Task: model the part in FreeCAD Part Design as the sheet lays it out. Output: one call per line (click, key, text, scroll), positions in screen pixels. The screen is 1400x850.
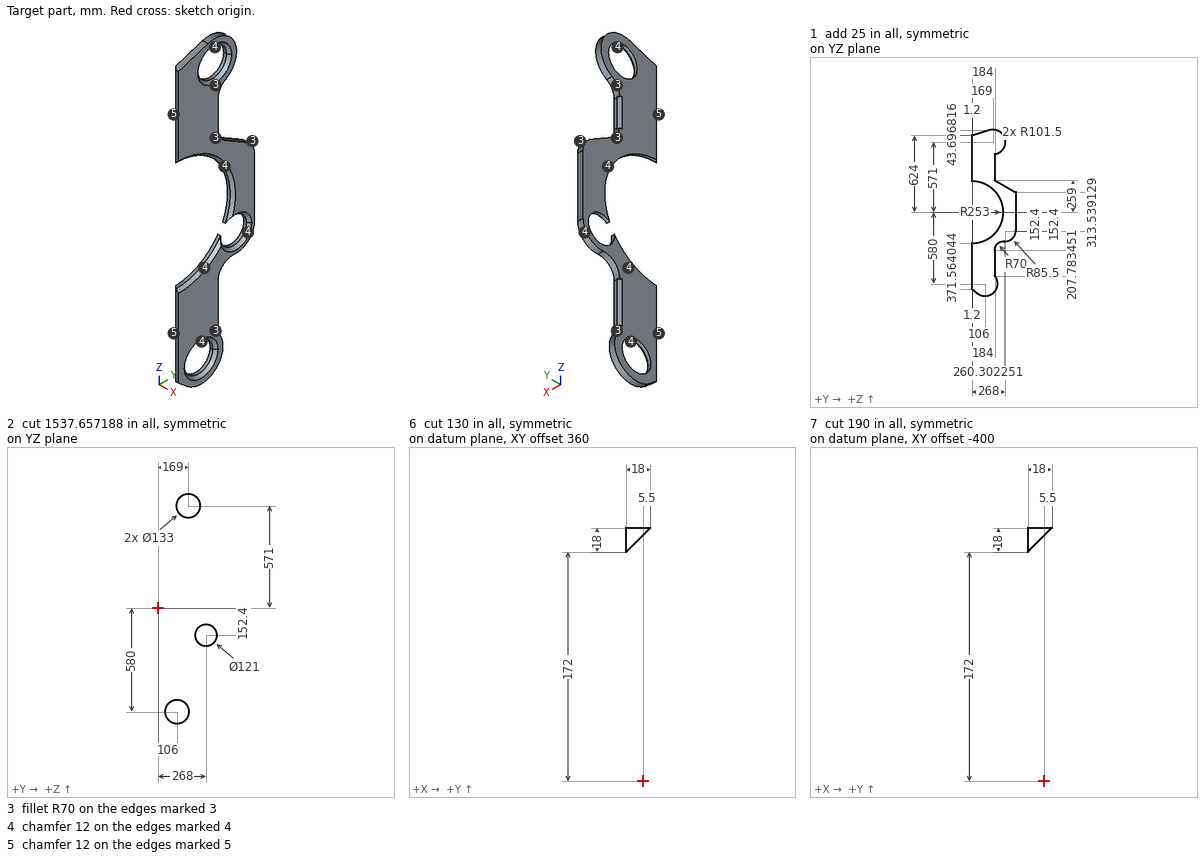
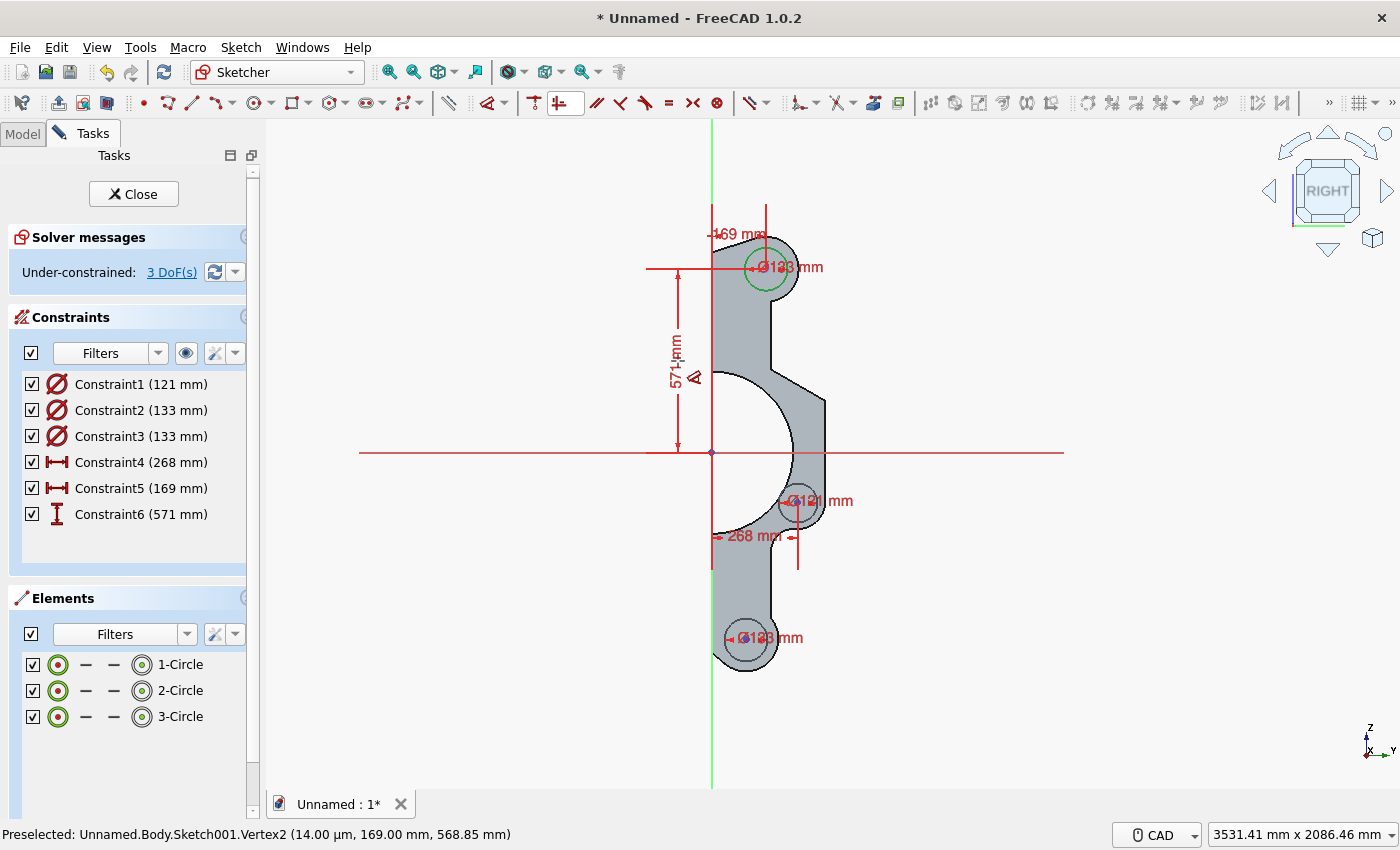
click(746, 640)
click(729, 674)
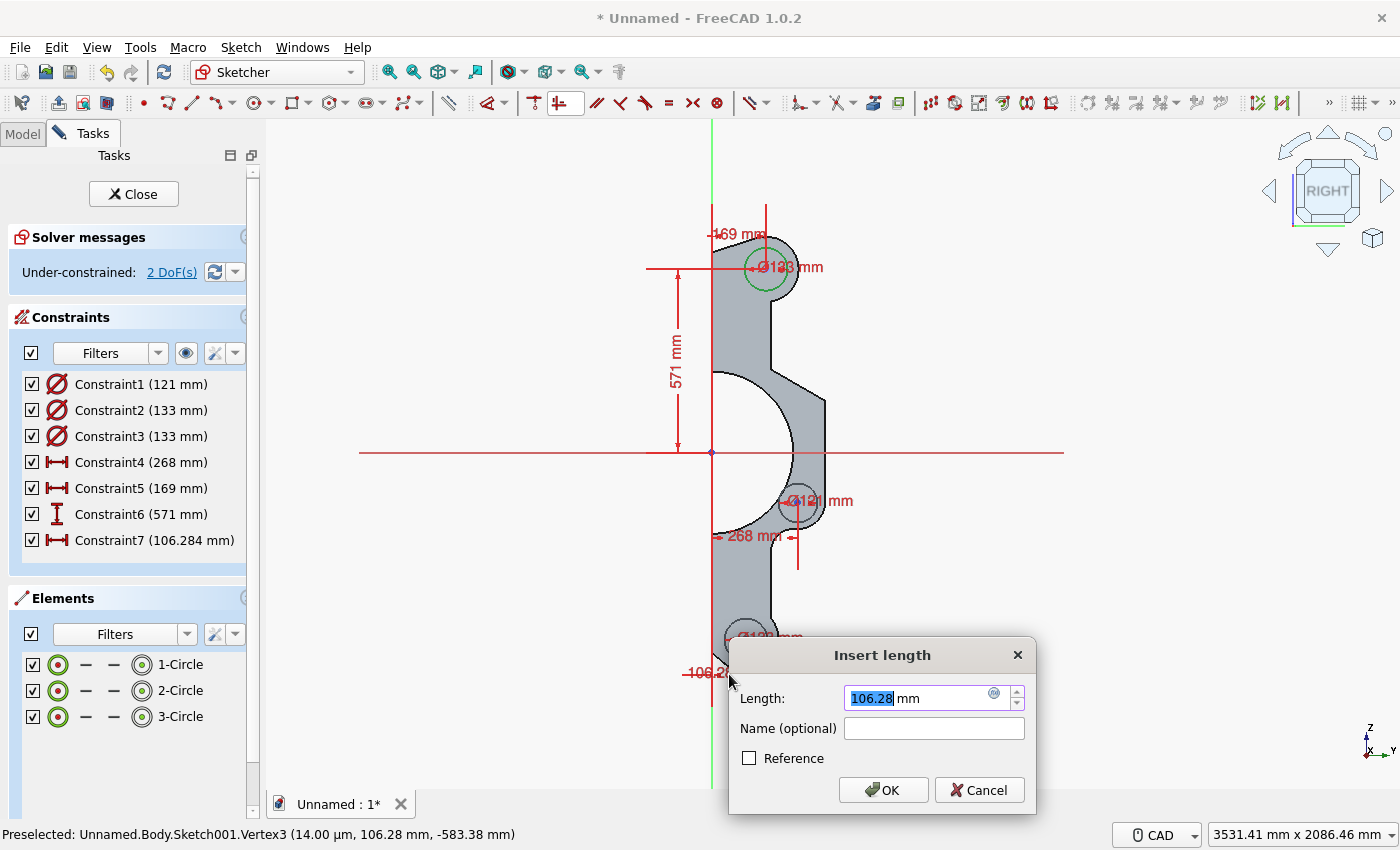
text(106)
key(Return)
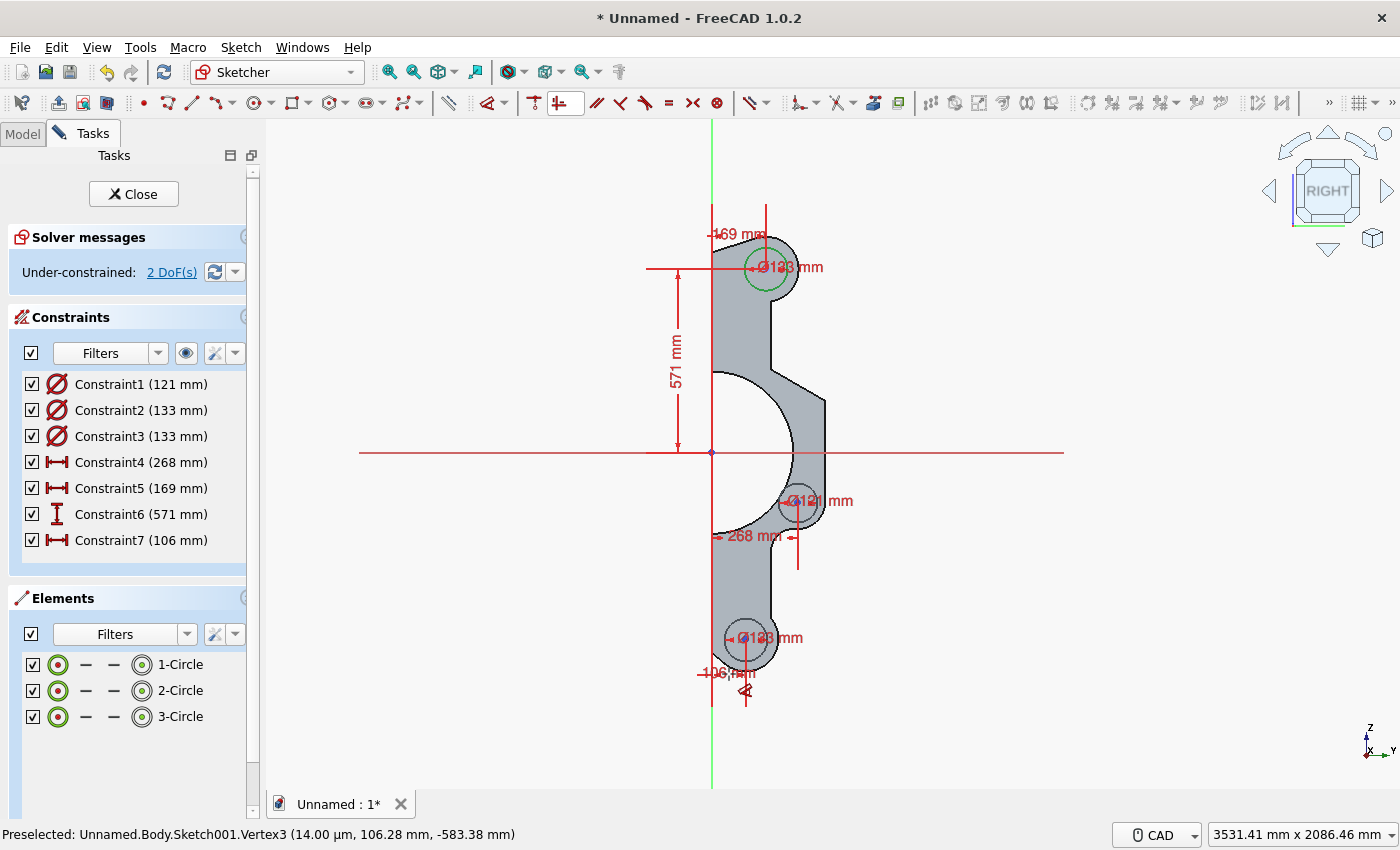
click(746, 640)
click(678, 546)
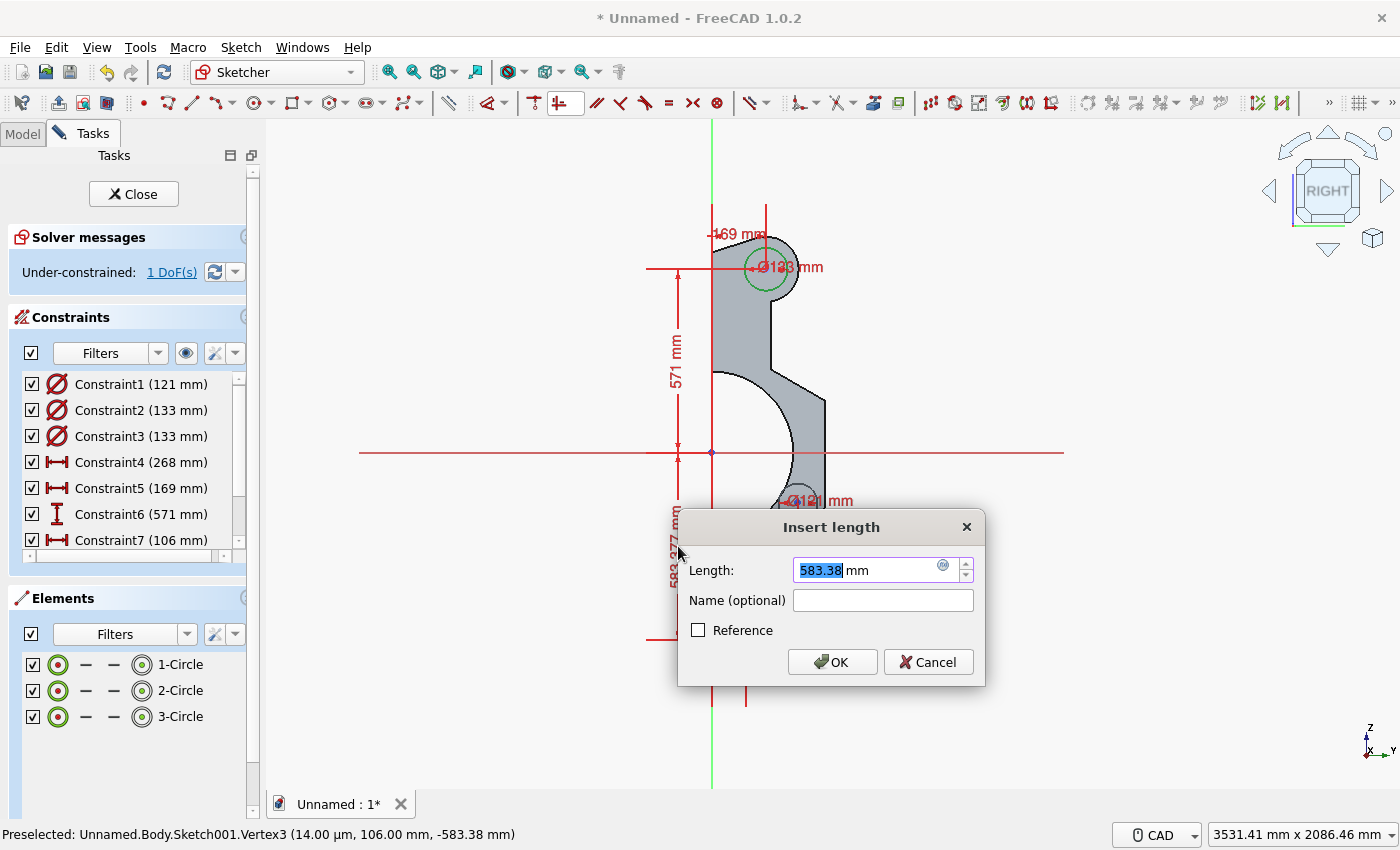
text(580)
key(Return)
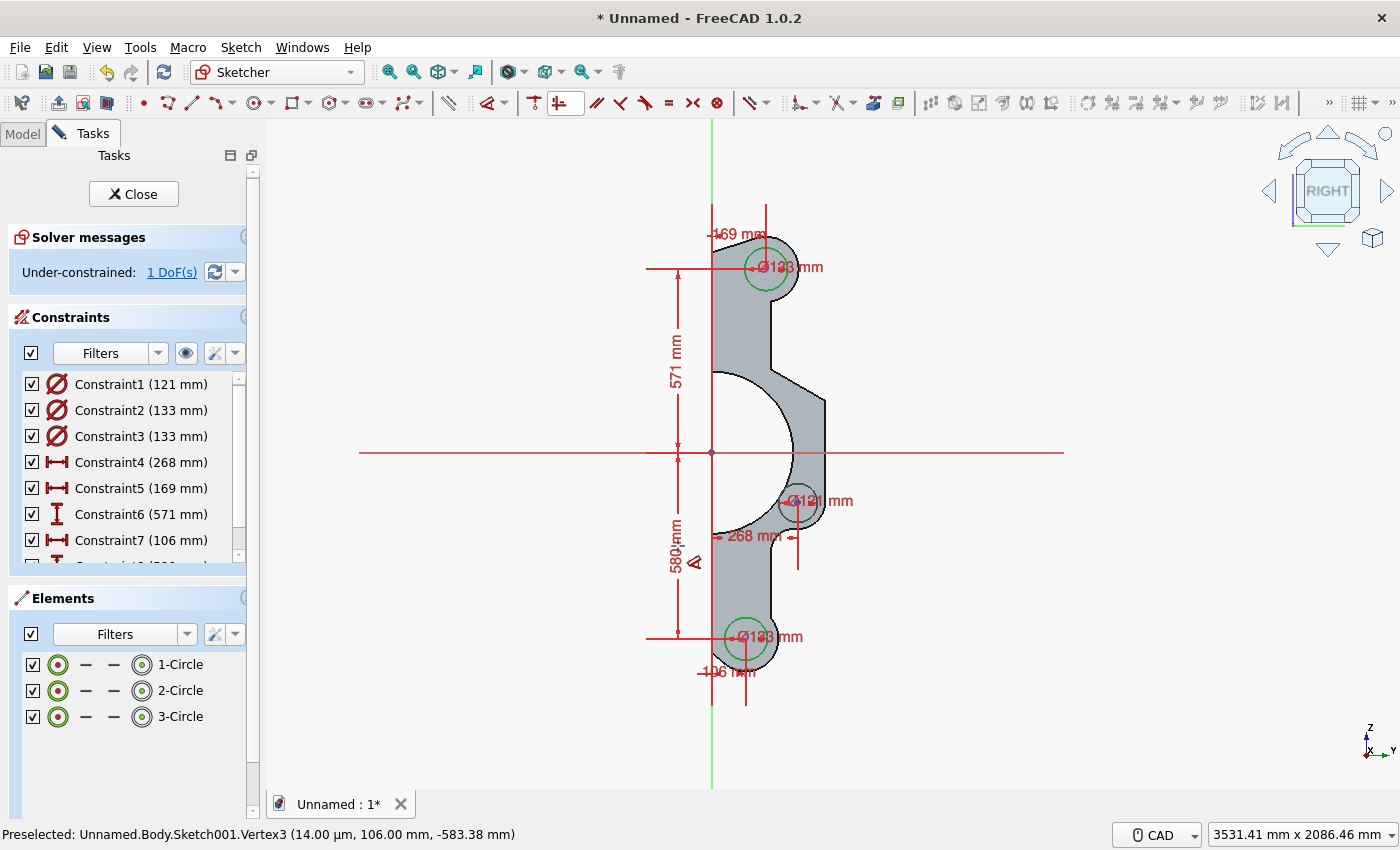
click(798, 503)
click(678, 478)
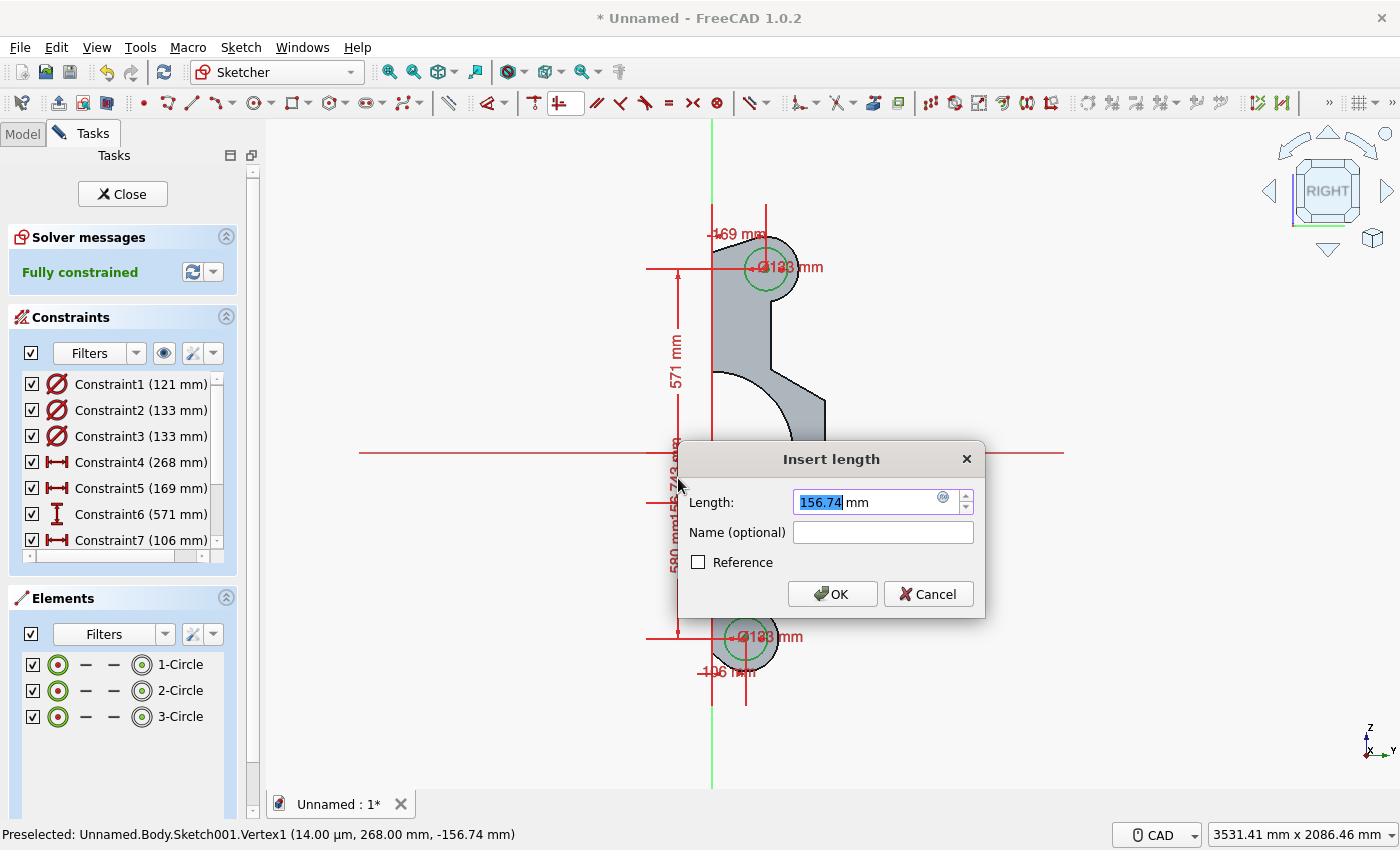
text(152.4)
key(Return)
key(Escape)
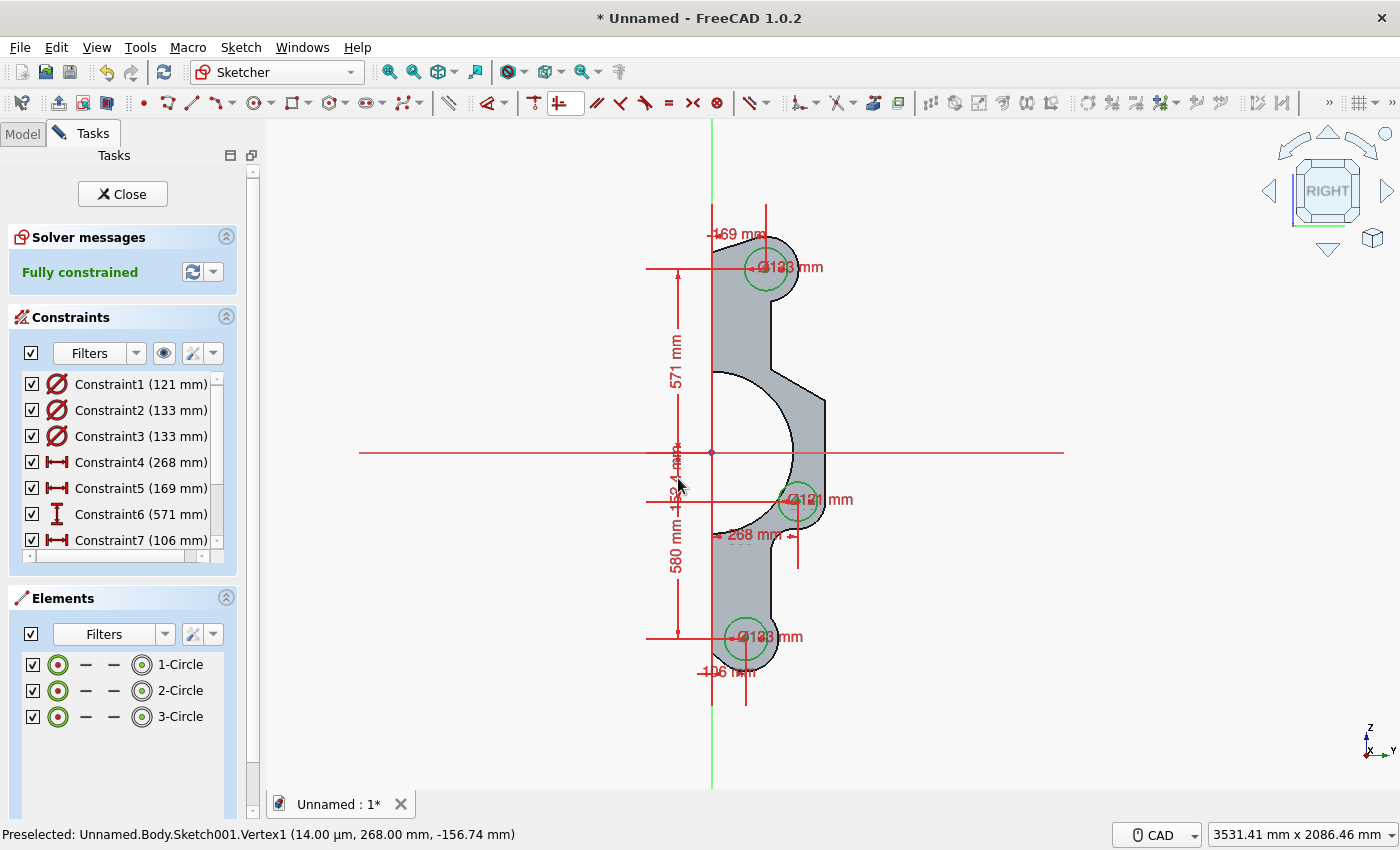
click(123, 194)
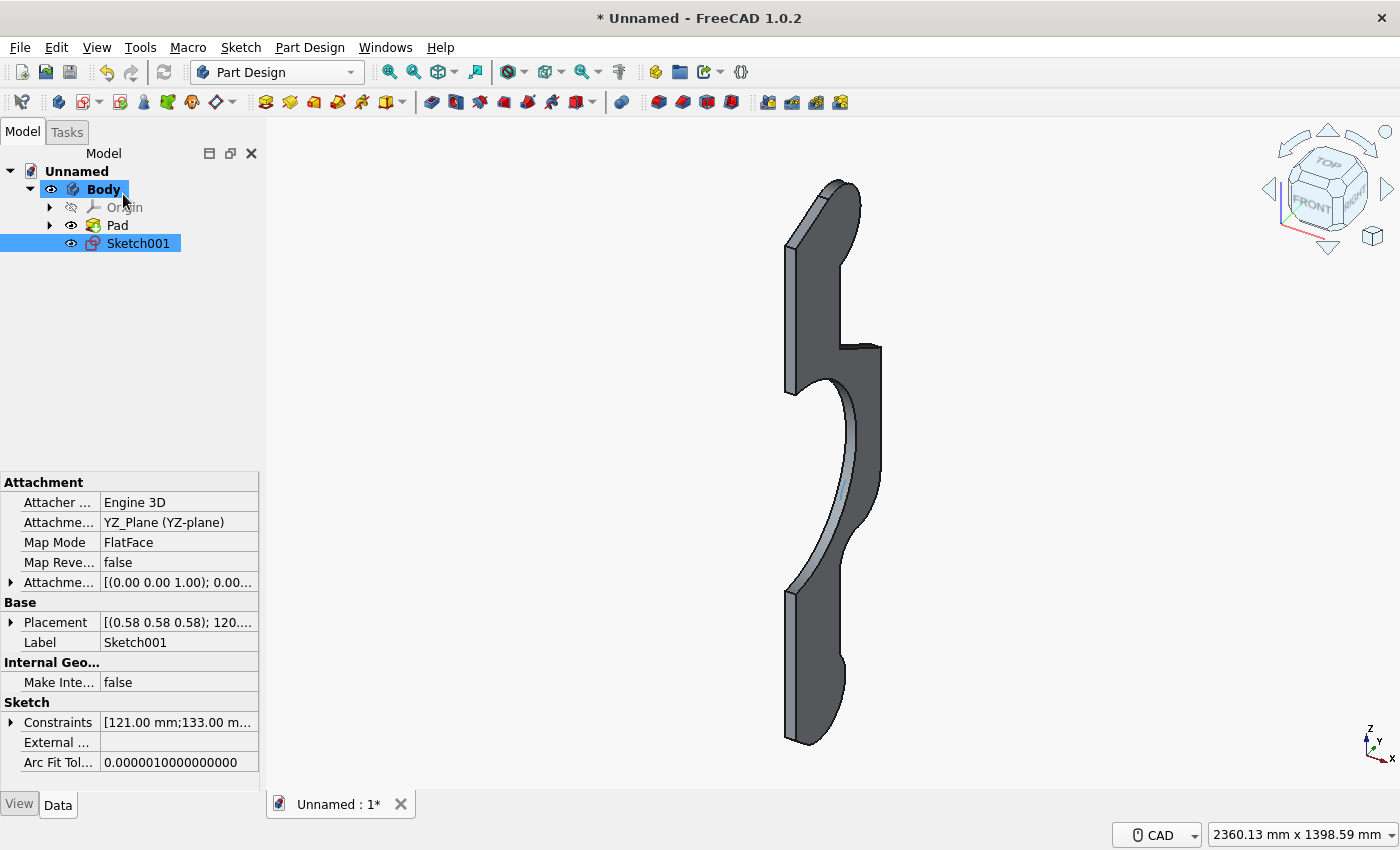
click(432, 102)